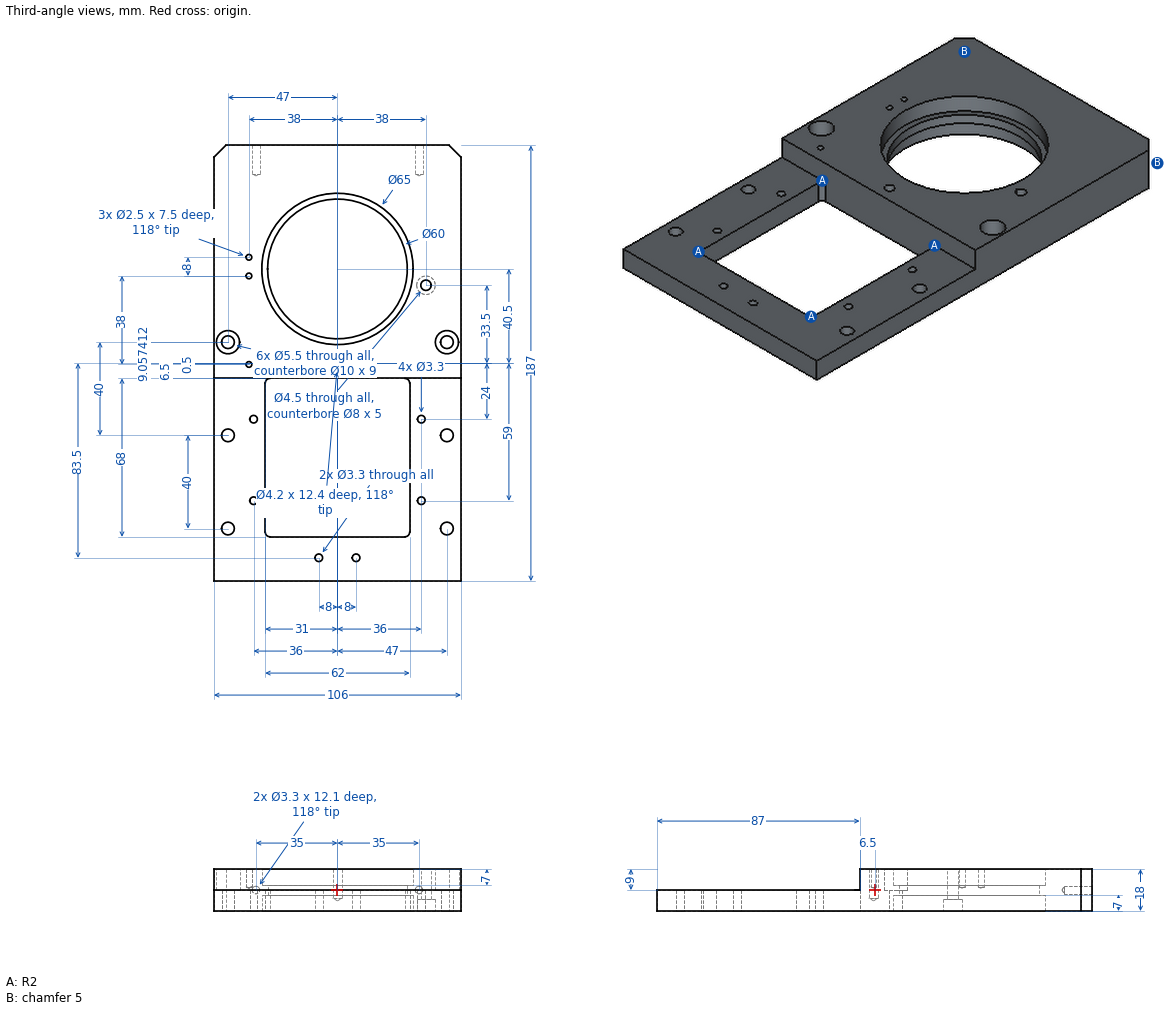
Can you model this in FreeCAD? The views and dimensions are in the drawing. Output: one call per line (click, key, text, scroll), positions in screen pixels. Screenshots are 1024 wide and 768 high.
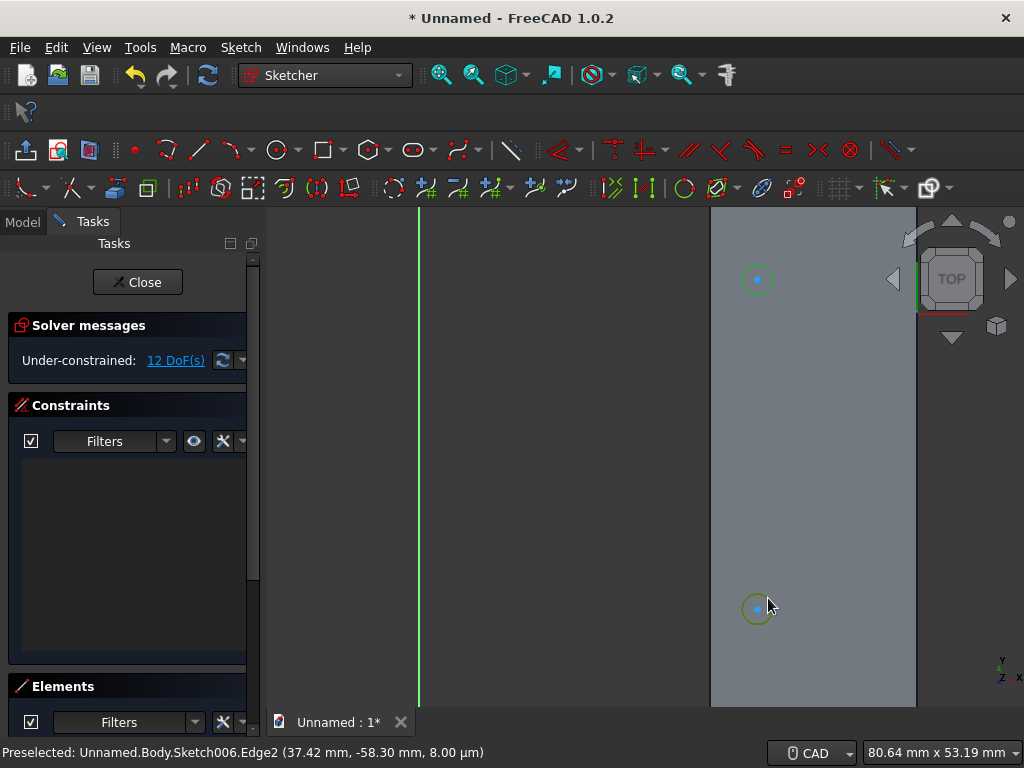
scroll(768, 601, down, 3)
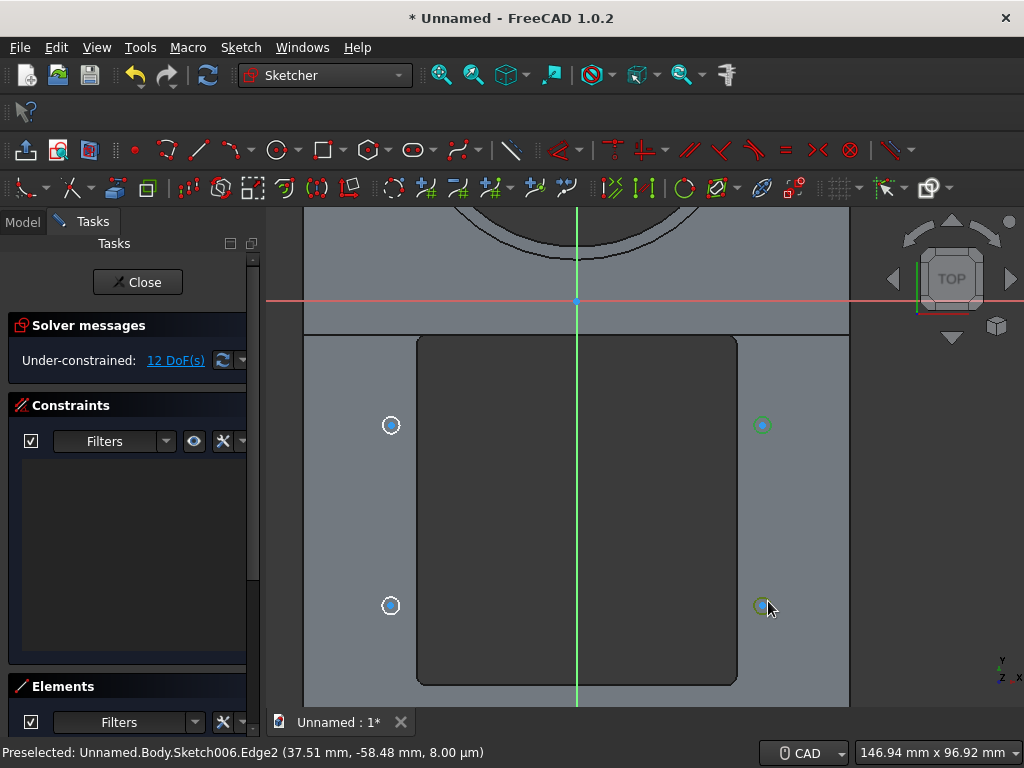
scroll(397, 600, up, 3)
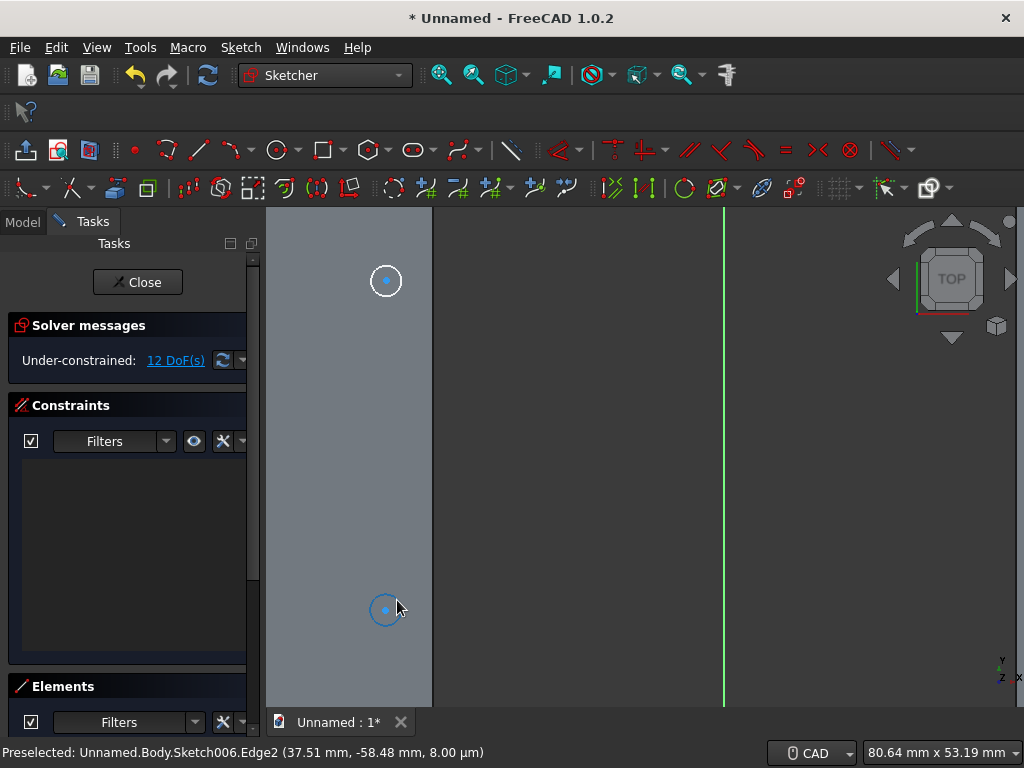
click(397, 599)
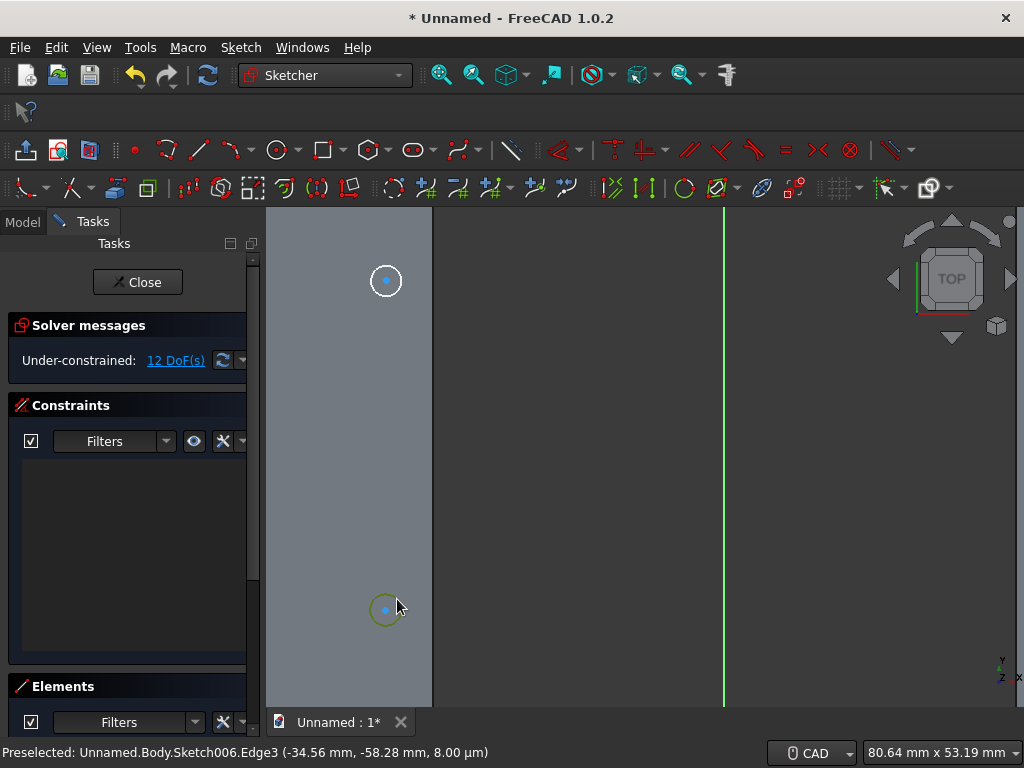
click(397, 270)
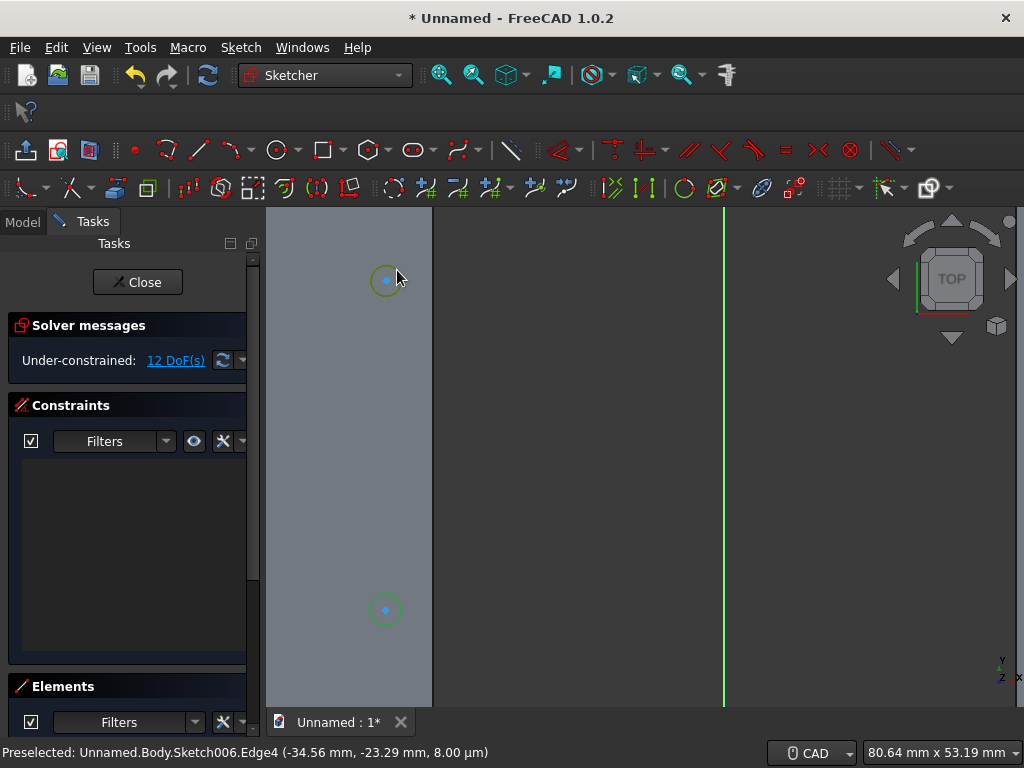
click(786, 150)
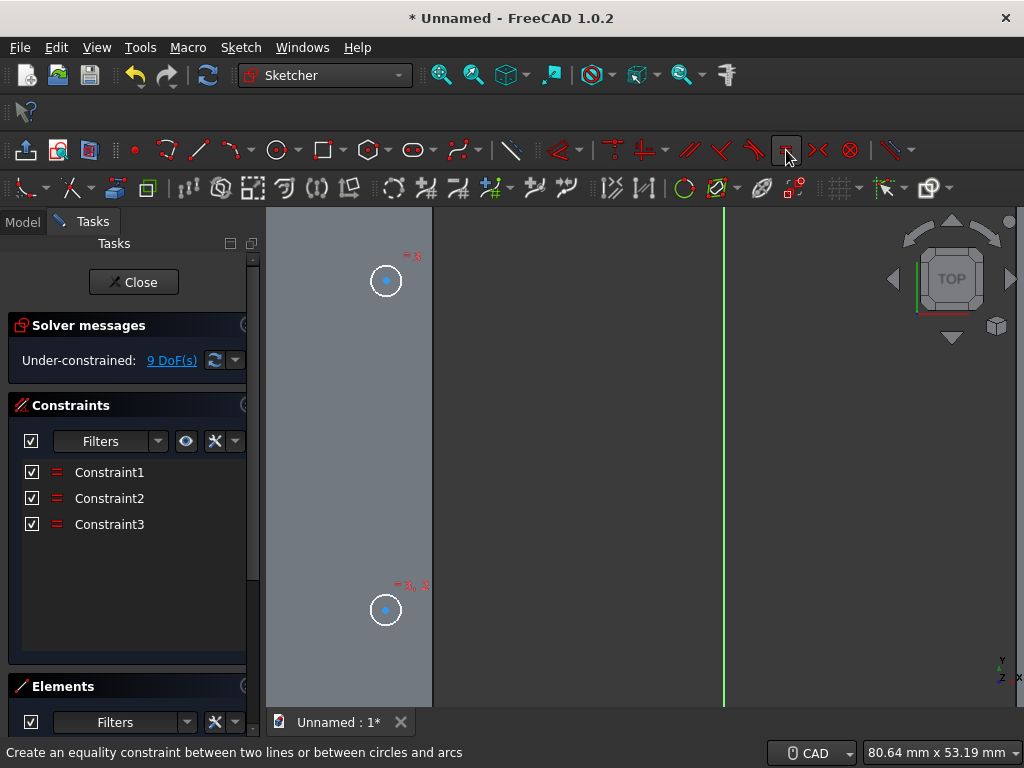
scroll(397, 600, down, 3)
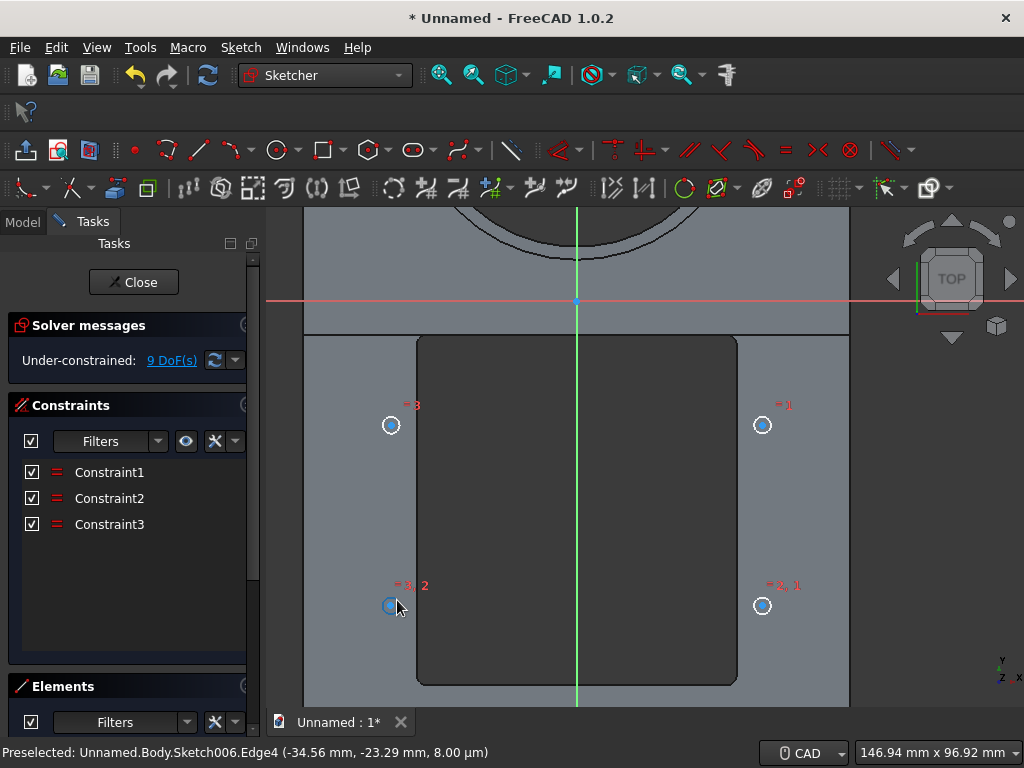
click(762, 425)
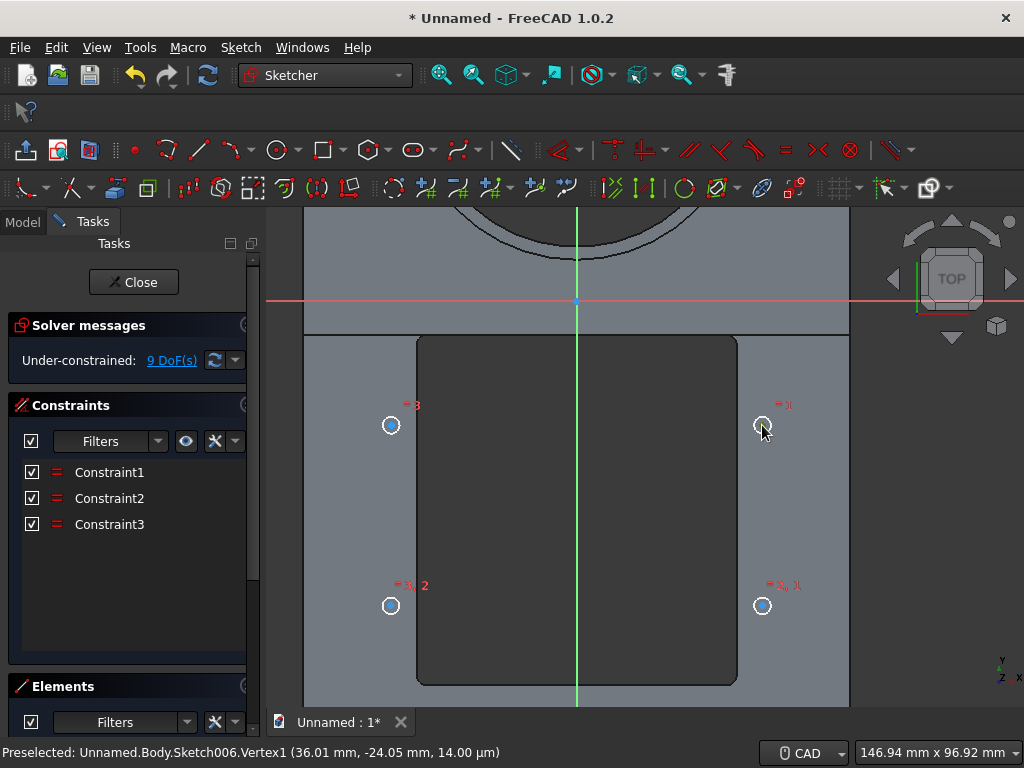
click(762, 606)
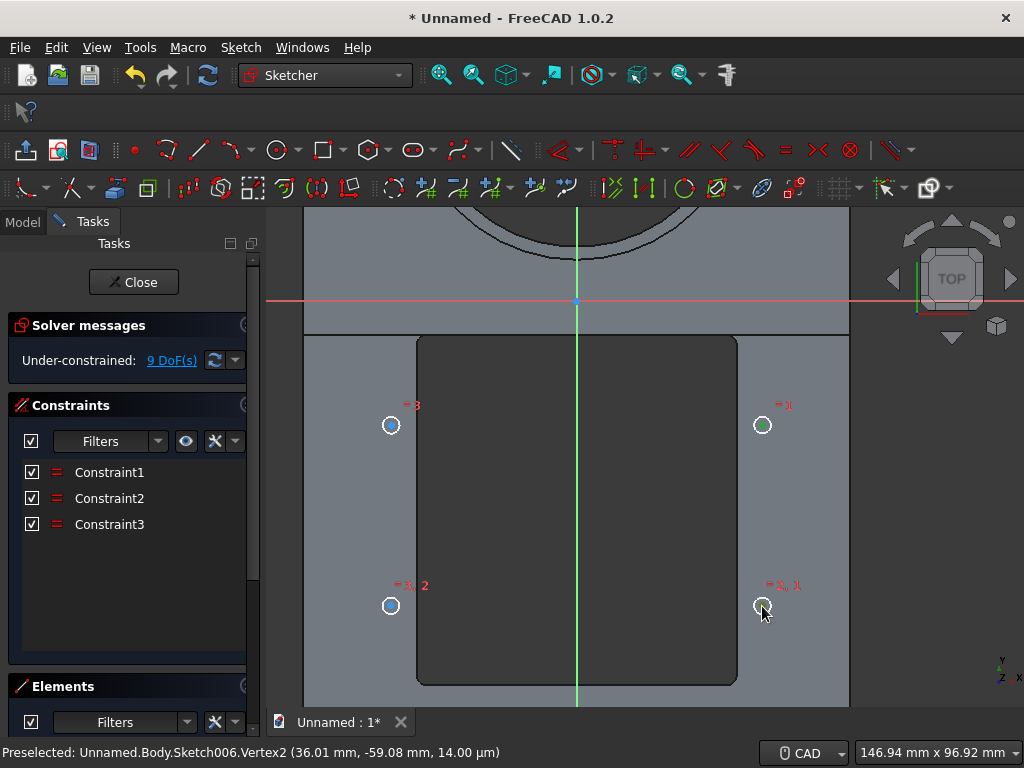
click(668, 150)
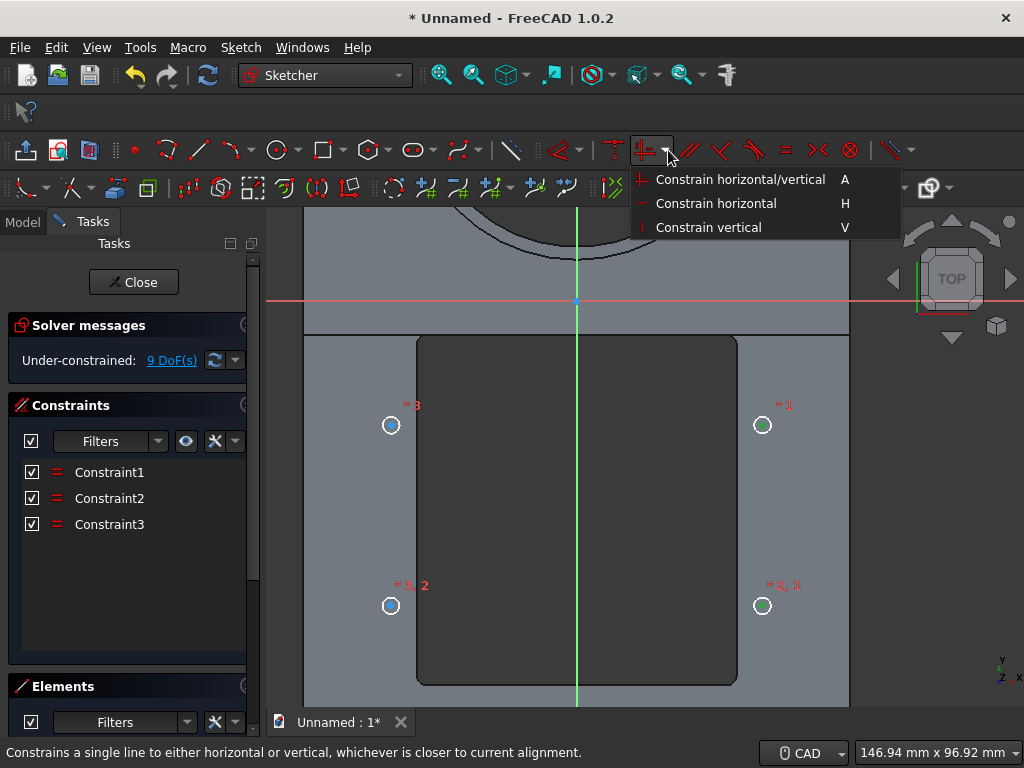
click(766, 227)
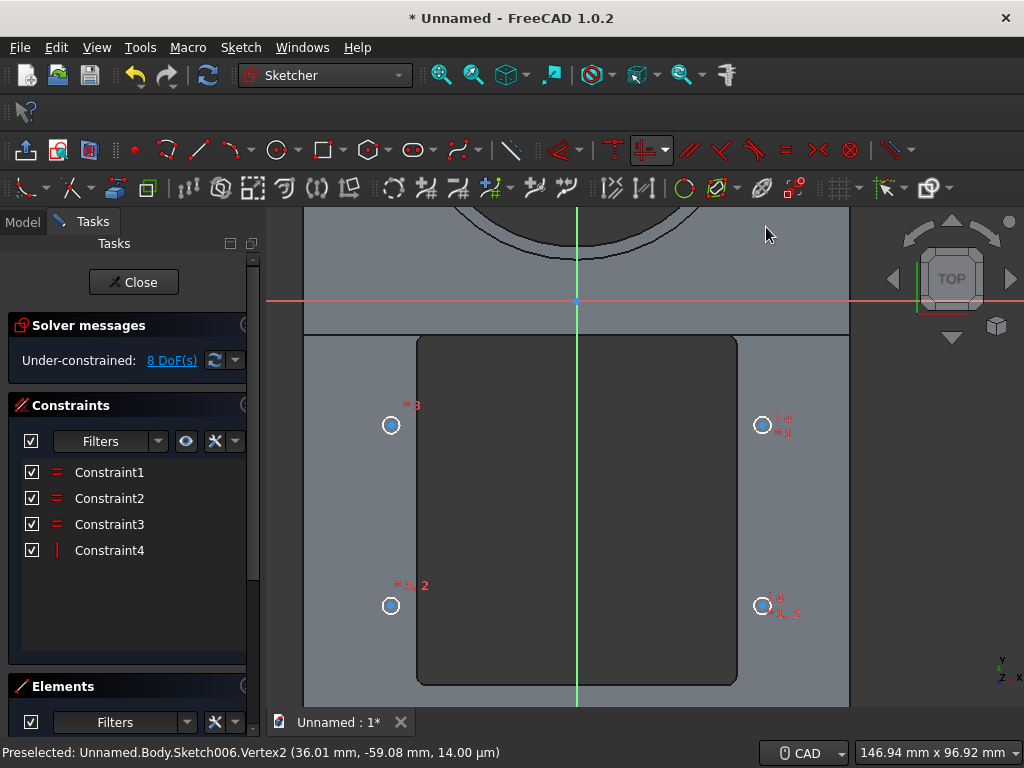
click(762, 606)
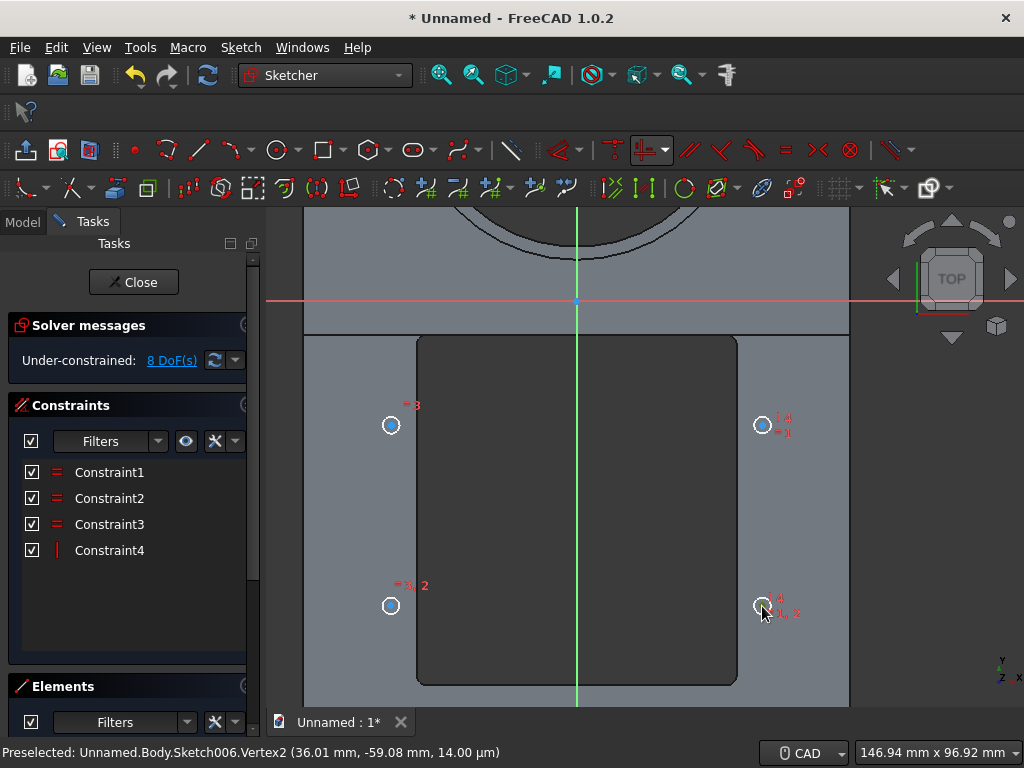
click(391, 606)